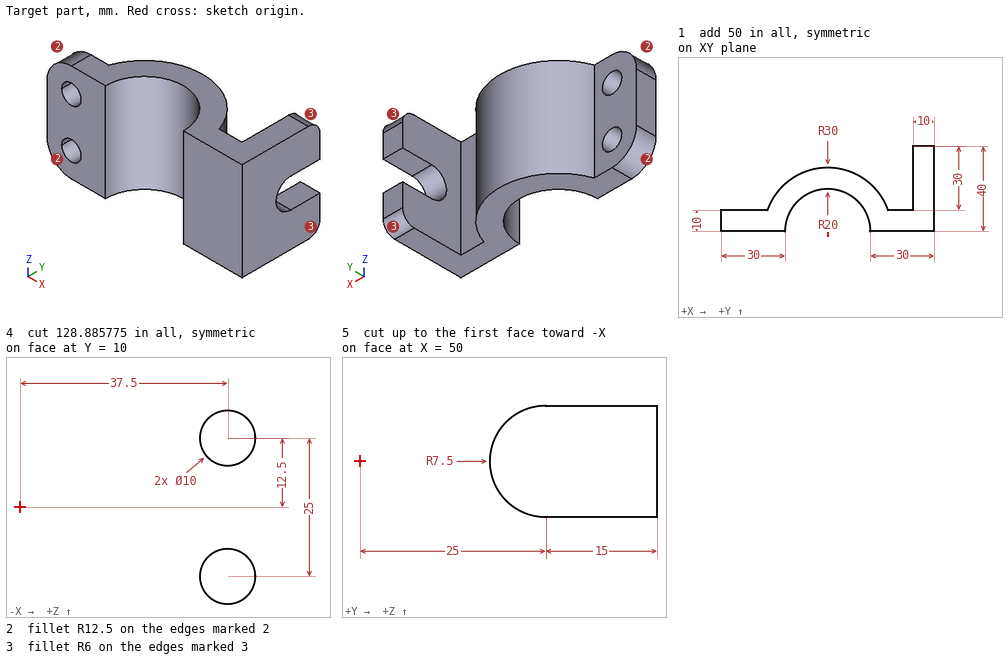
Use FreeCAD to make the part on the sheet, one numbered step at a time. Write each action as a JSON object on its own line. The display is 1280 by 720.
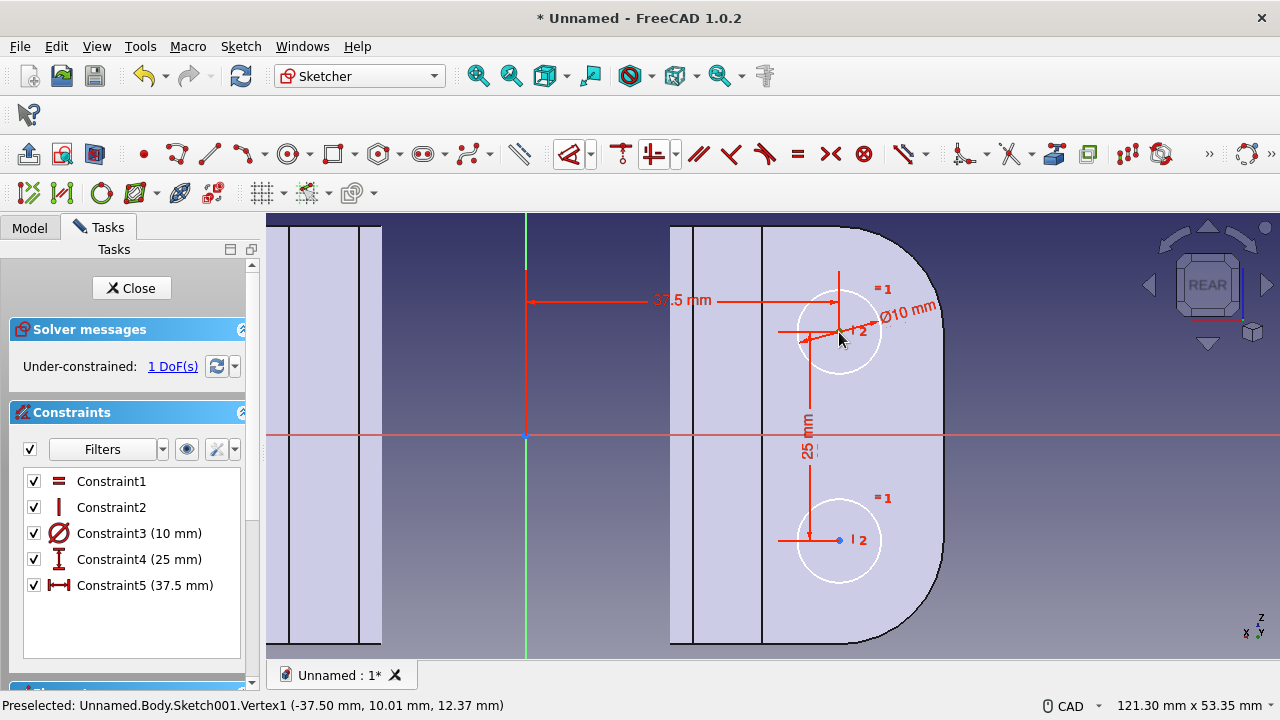
{"action": "key", "text": "i"}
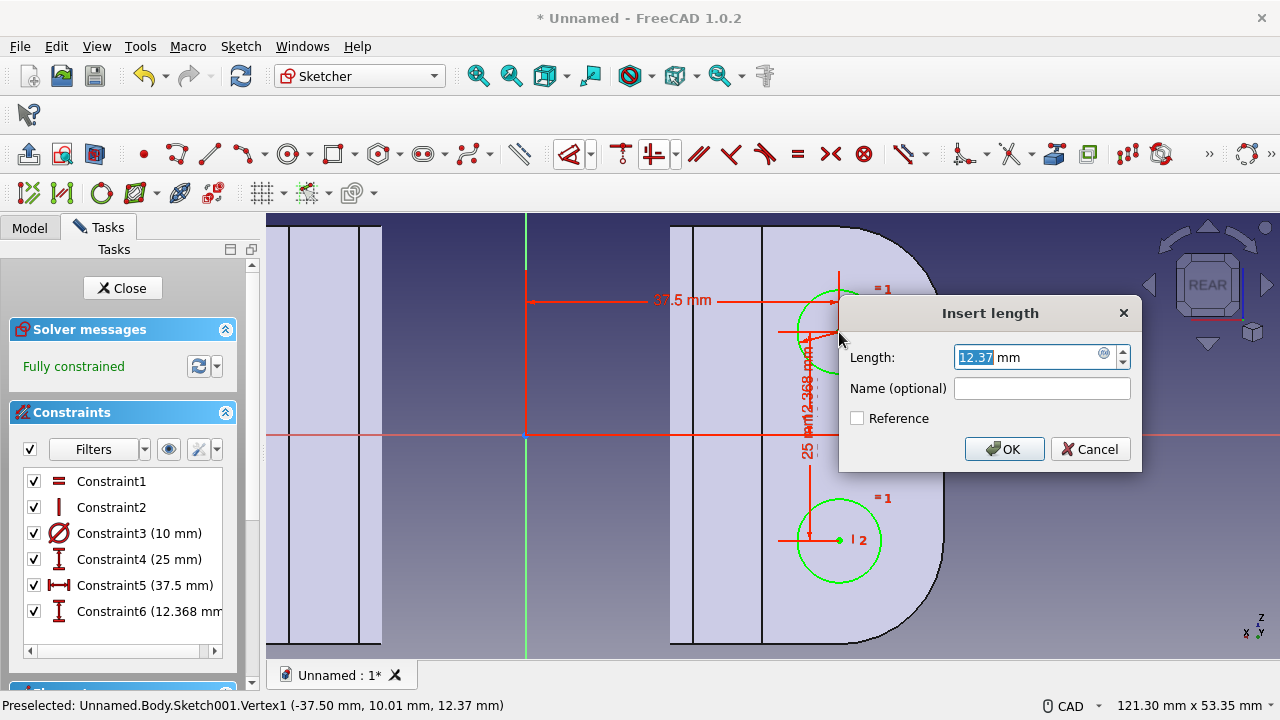
{"action": "type", "text": "12.5"}
{"action": "key", "text": "Return"}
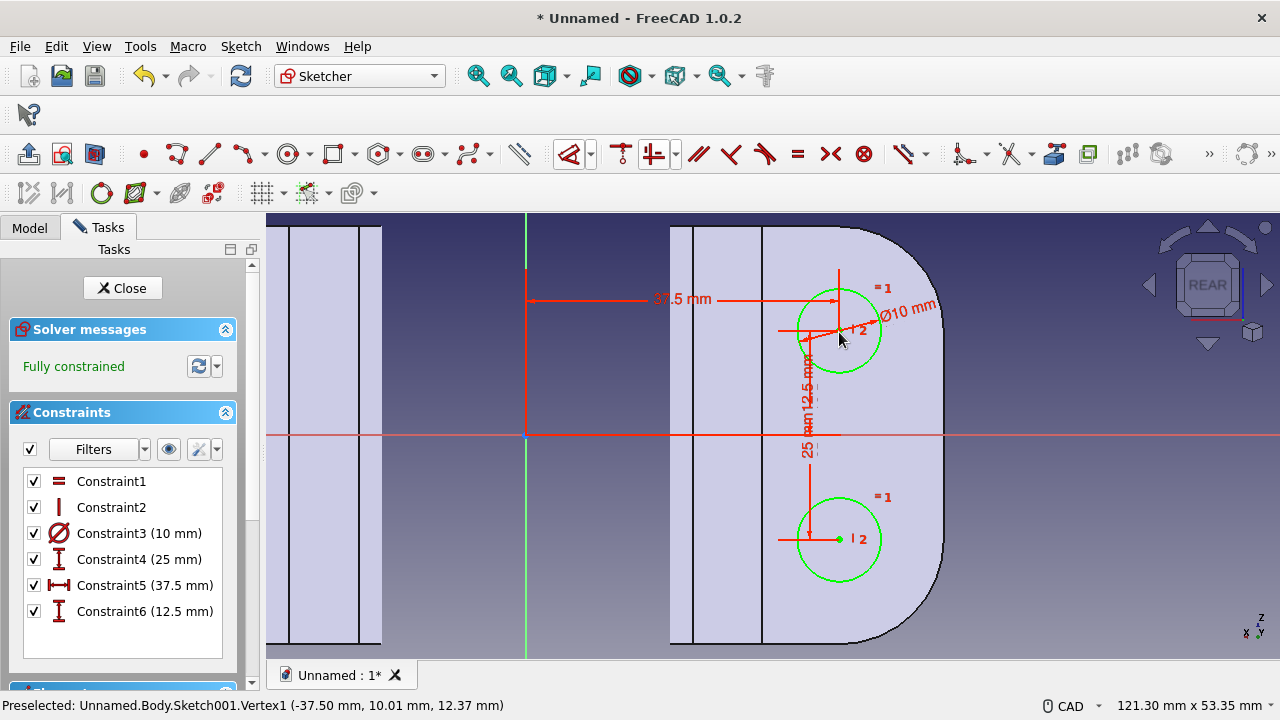
{"action": "left_click", "coordinate": [123, 288]}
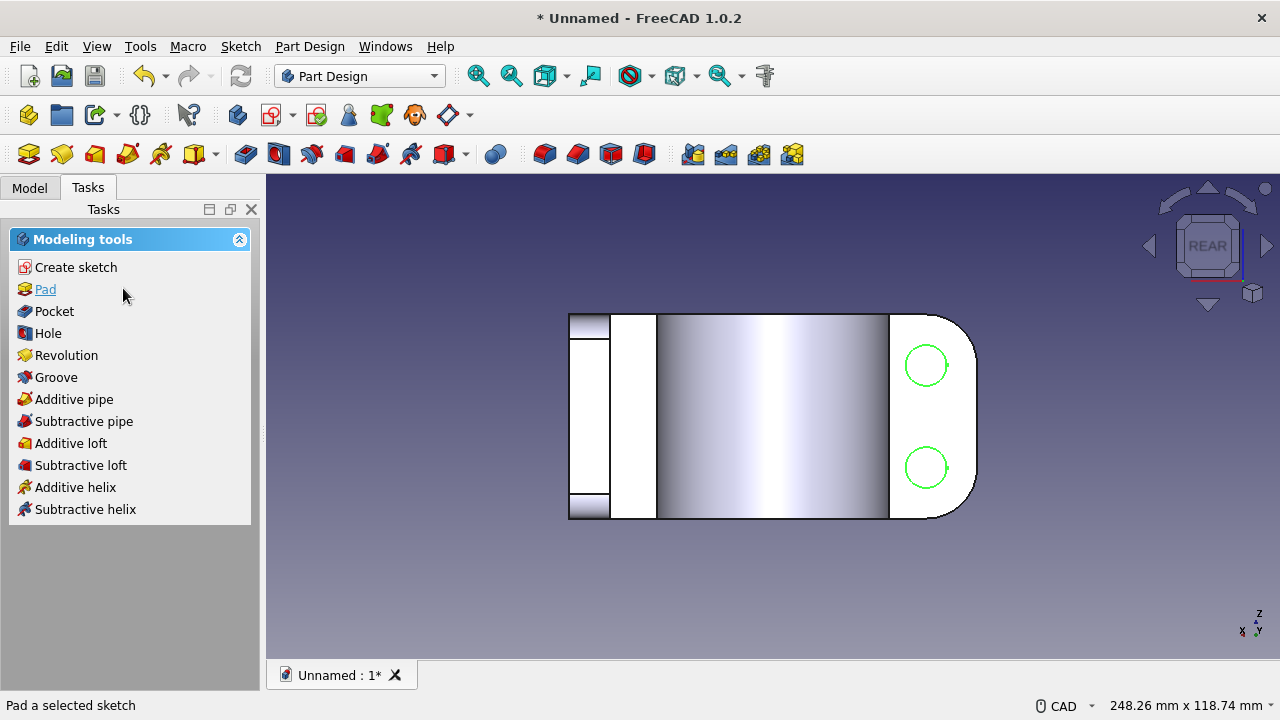
{"action": "left_click", "coordinate": [246, 154]}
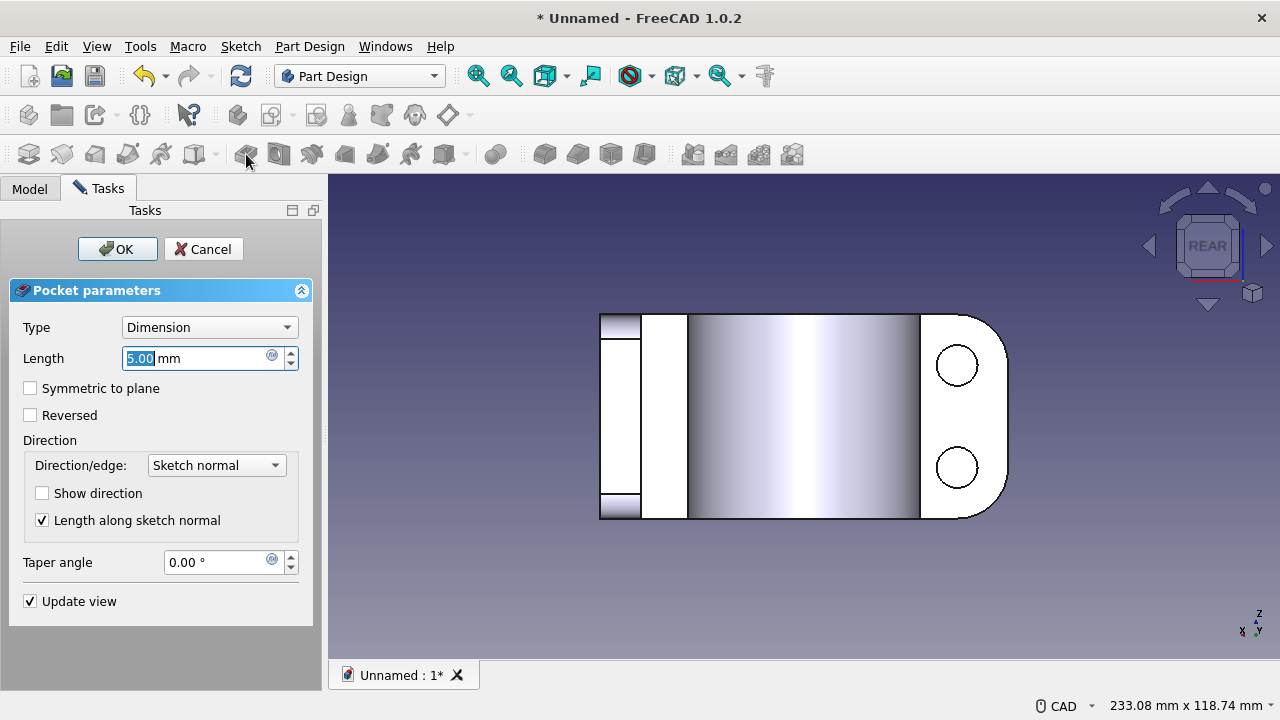
{"action": "type", "text": "128.885775"}
{"action": "key", "text": "Tab"}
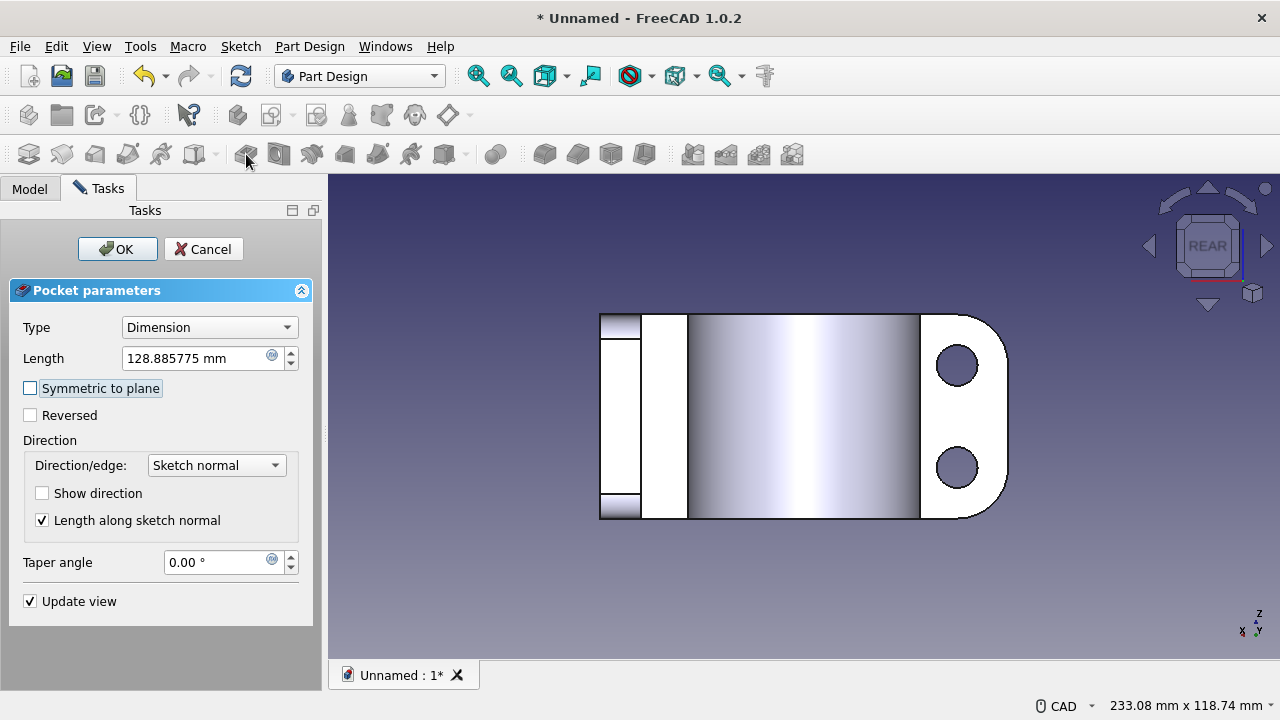
{"action": "left_click", "coordinate": [31, 388]}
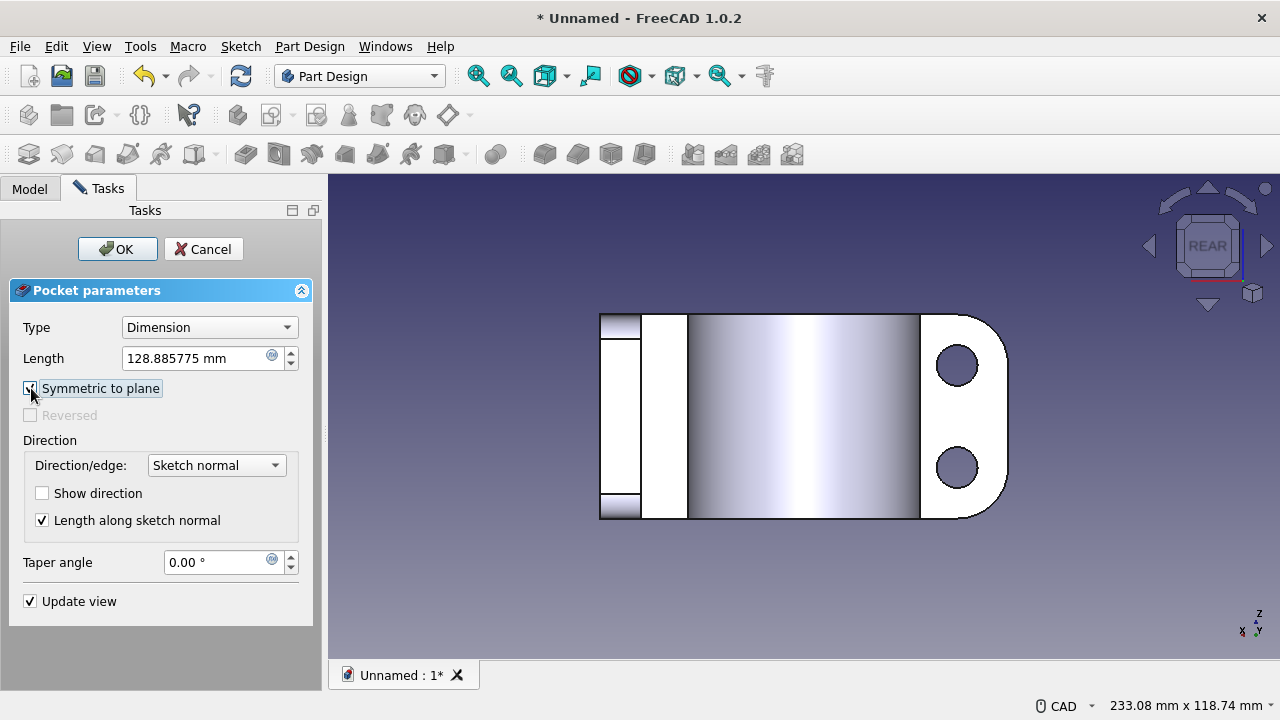
{"action": "left_click", "coordinate": [118, 249]}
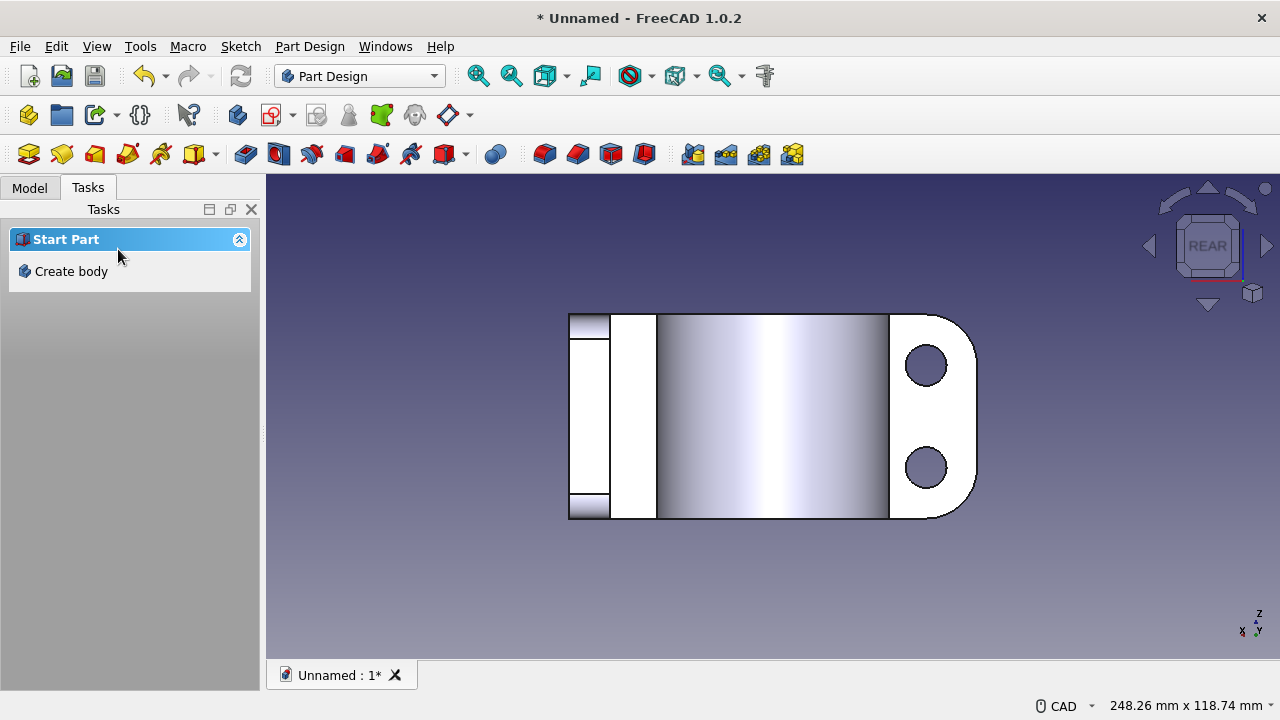
{"action": "left_click", "coordinate": [479, 76]}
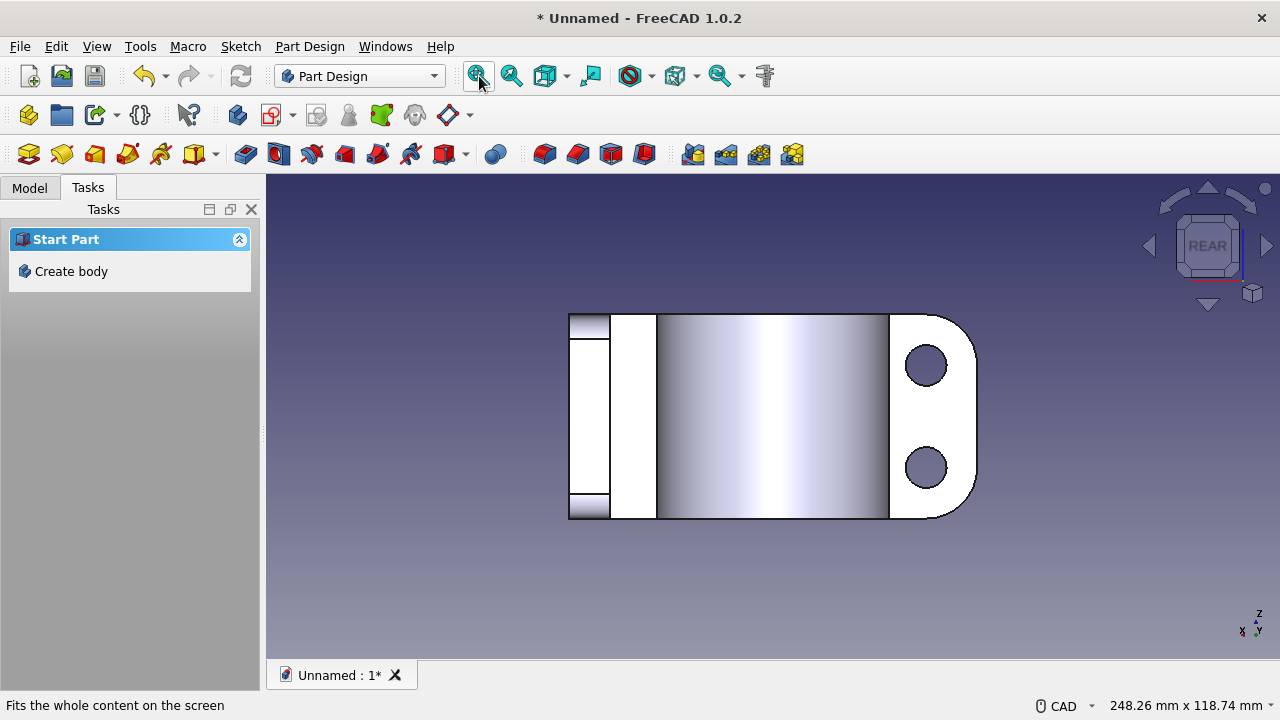
{"action": "key", "text": "0"}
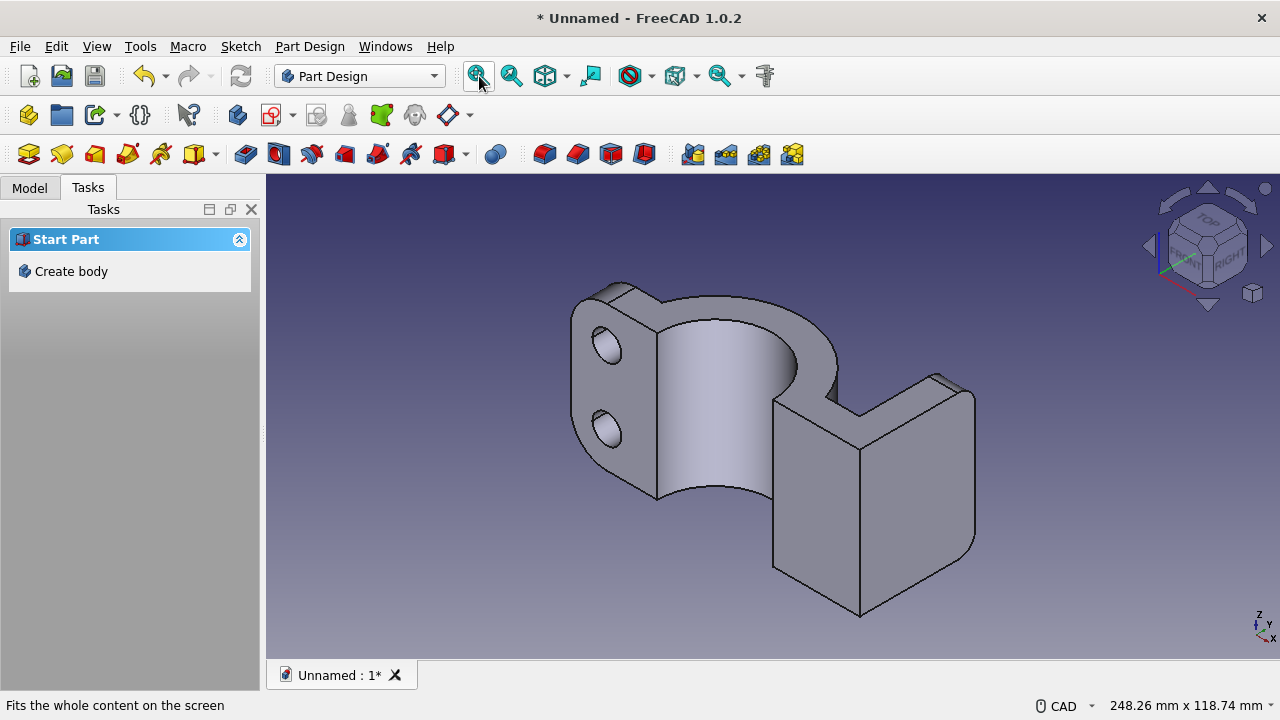
{"action": "left_click", "coordinate": [917, 499]}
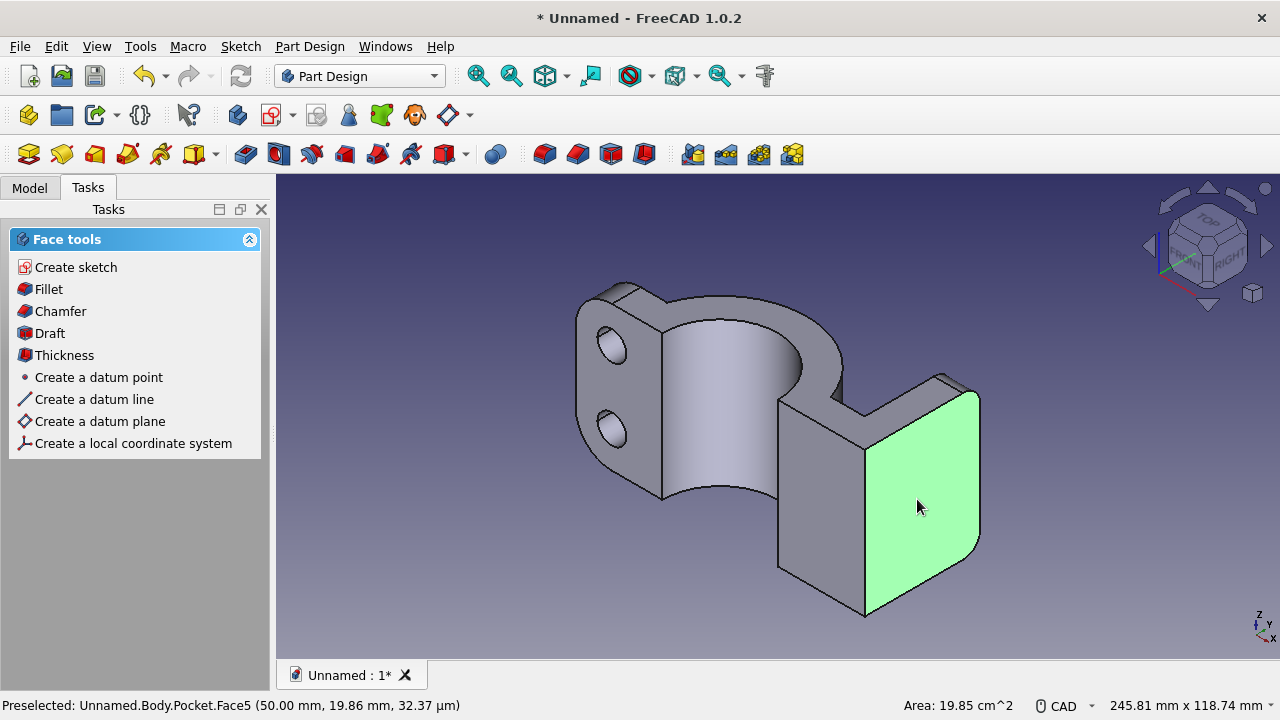
{"action": "left_click", "coordinate": [270, 116]}